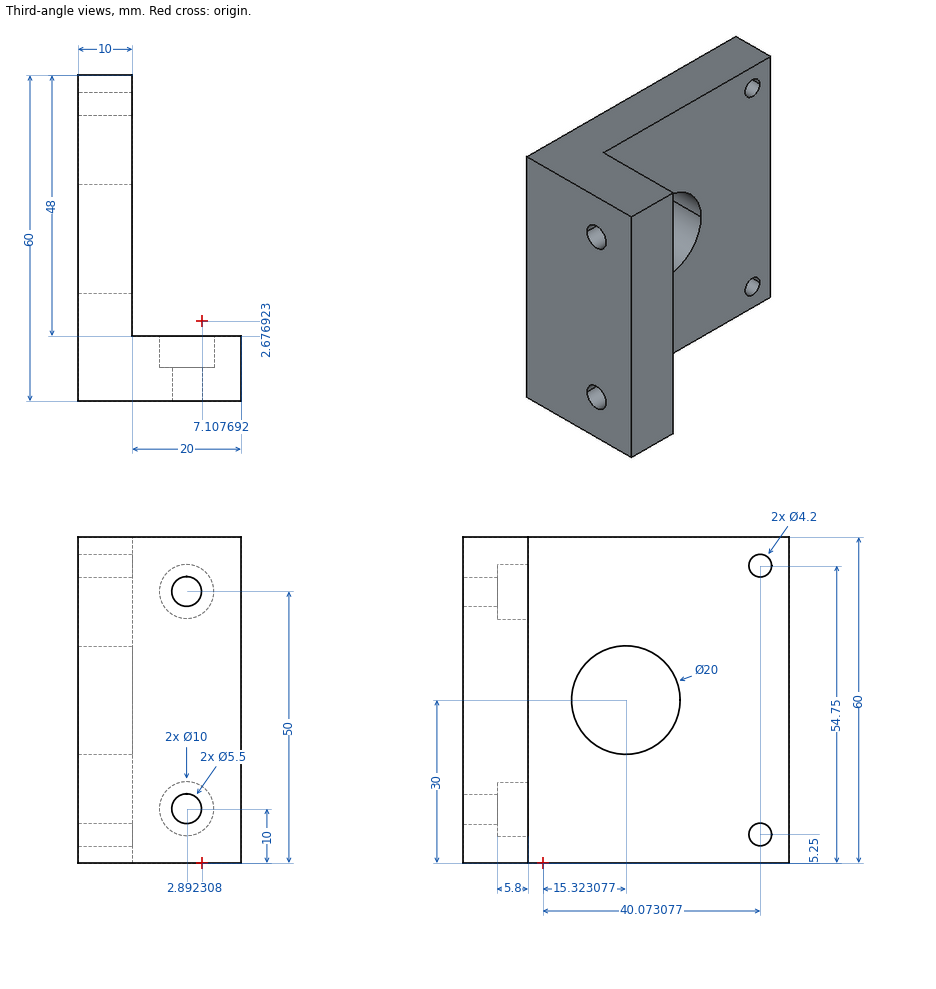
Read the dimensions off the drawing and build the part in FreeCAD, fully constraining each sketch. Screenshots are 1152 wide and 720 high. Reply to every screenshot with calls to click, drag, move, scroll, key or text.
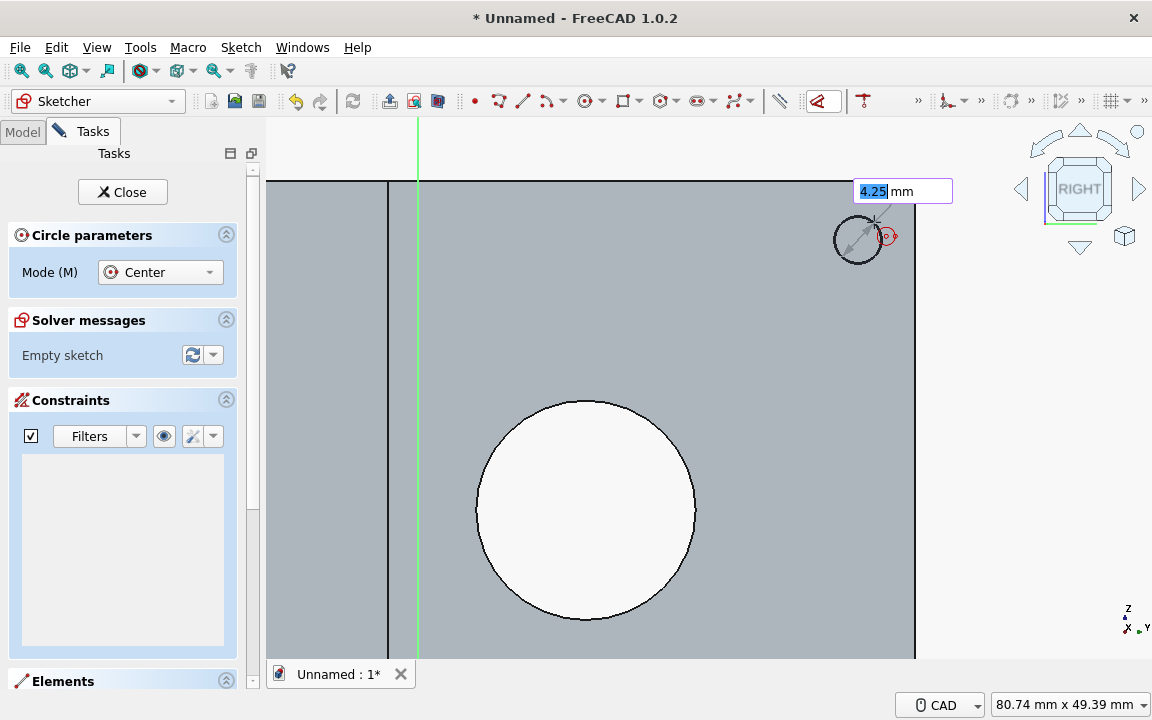
text(4.2)
key(Return)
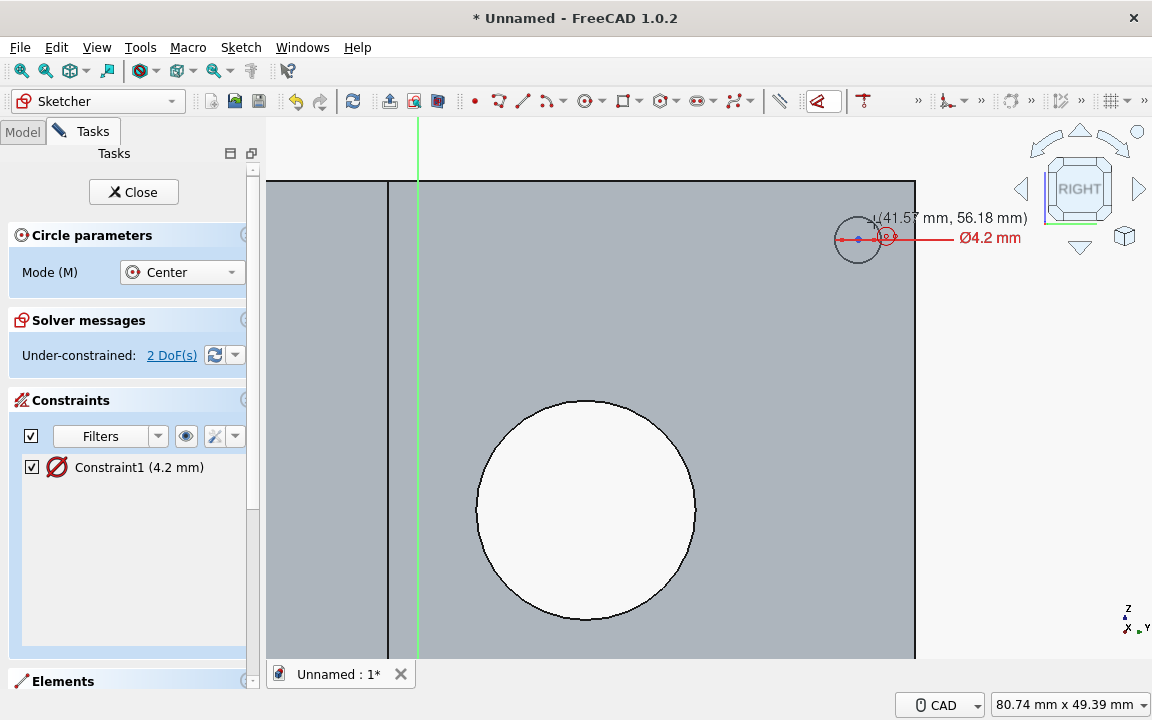
scroll(630, 218, down, 3)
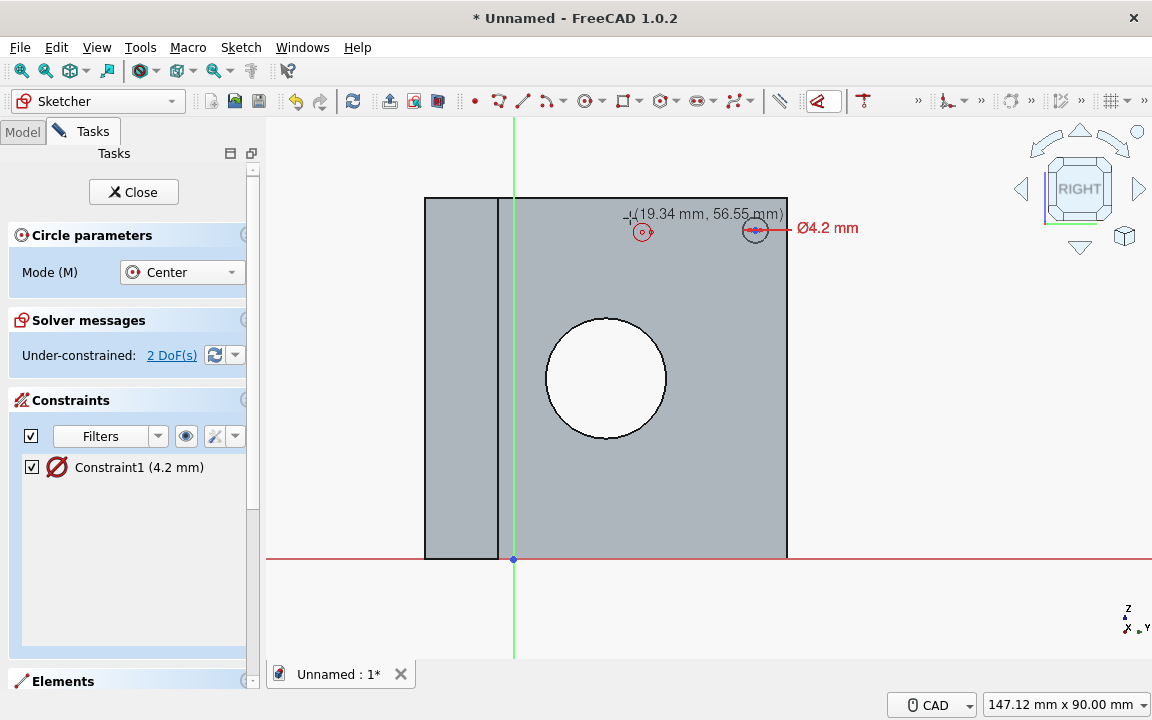
scroll(755, 528, up, 3)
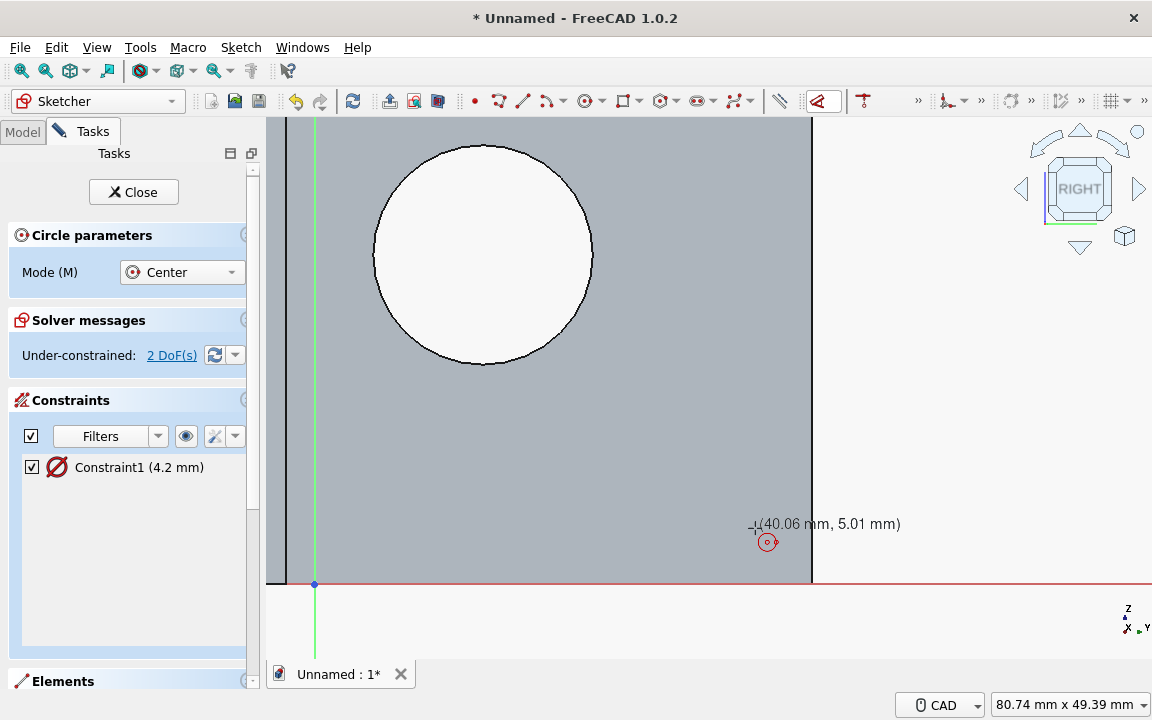
click(755, 527)
move(771, 510)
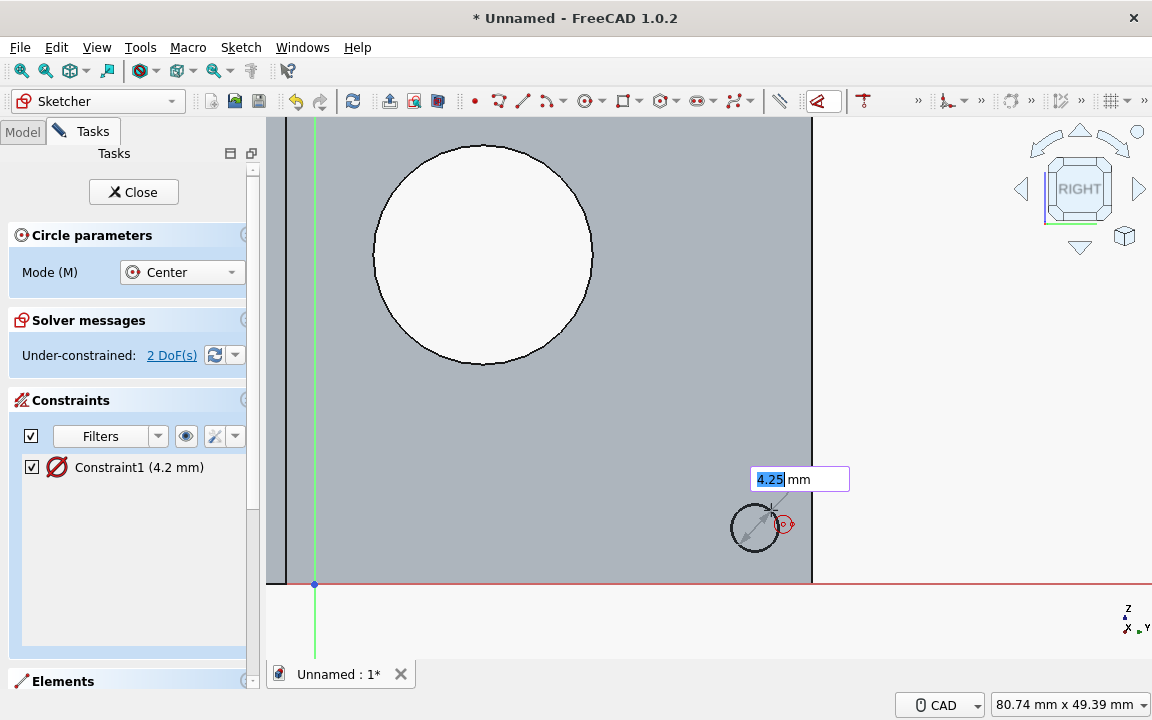
text(4.2)
key(Return)
key(Escape)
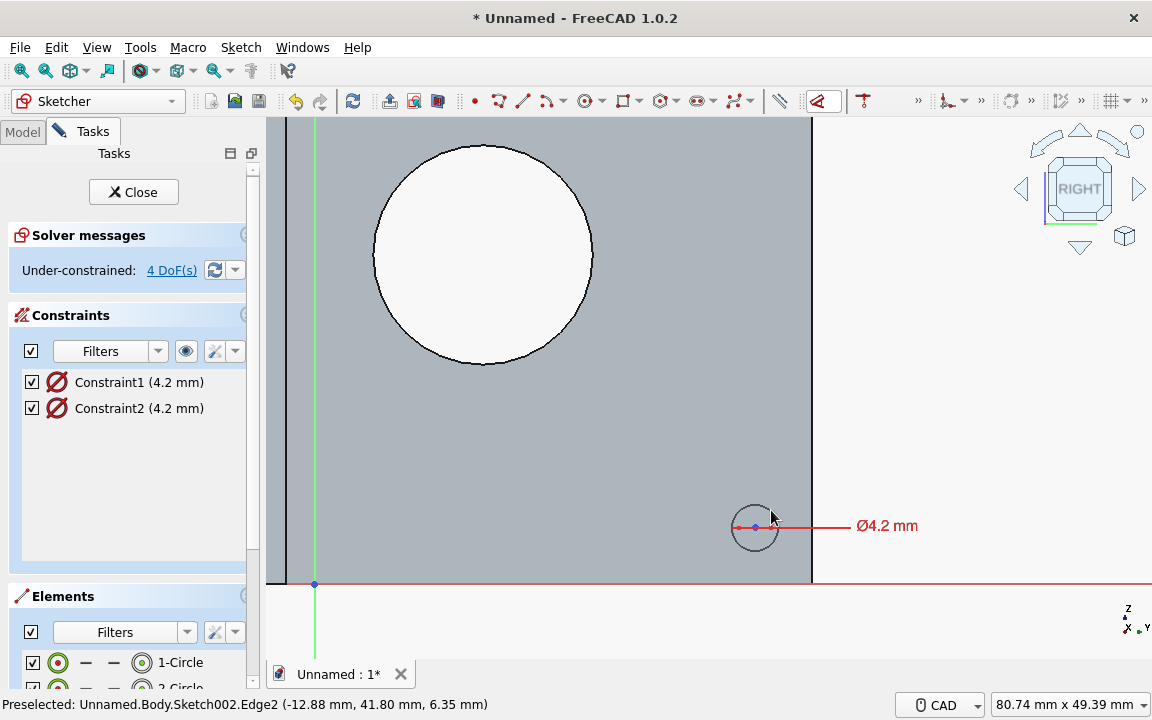
scroll(755, 529, down, 3)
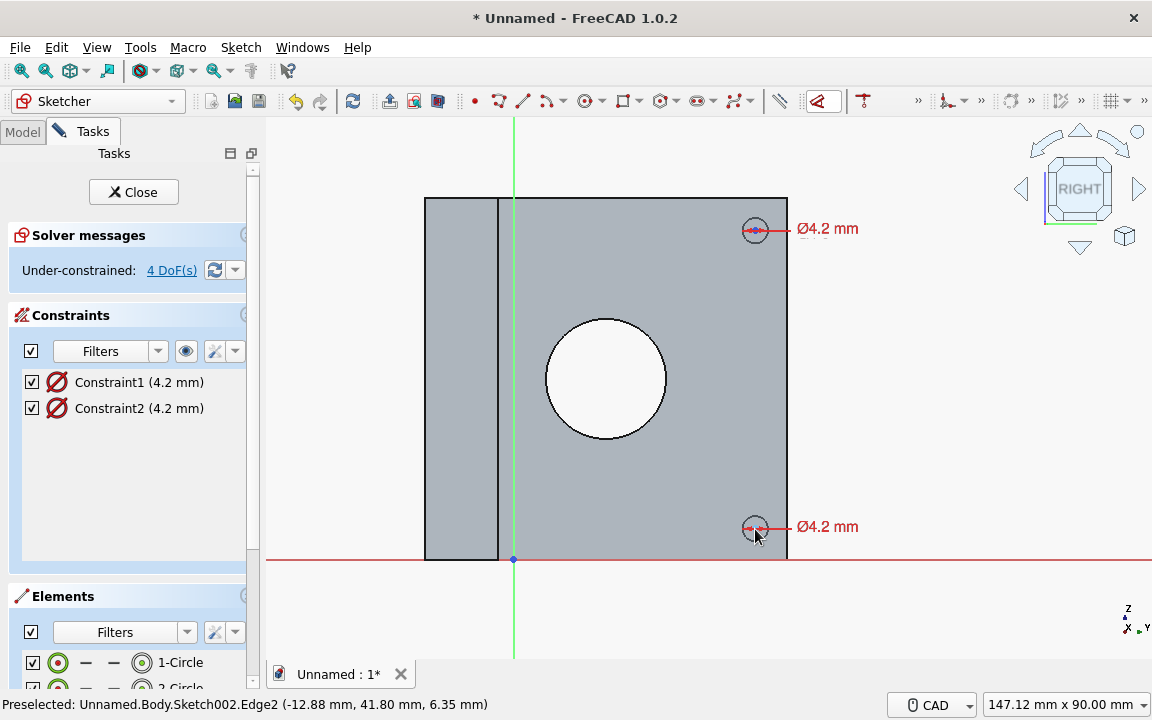
click(755, 231)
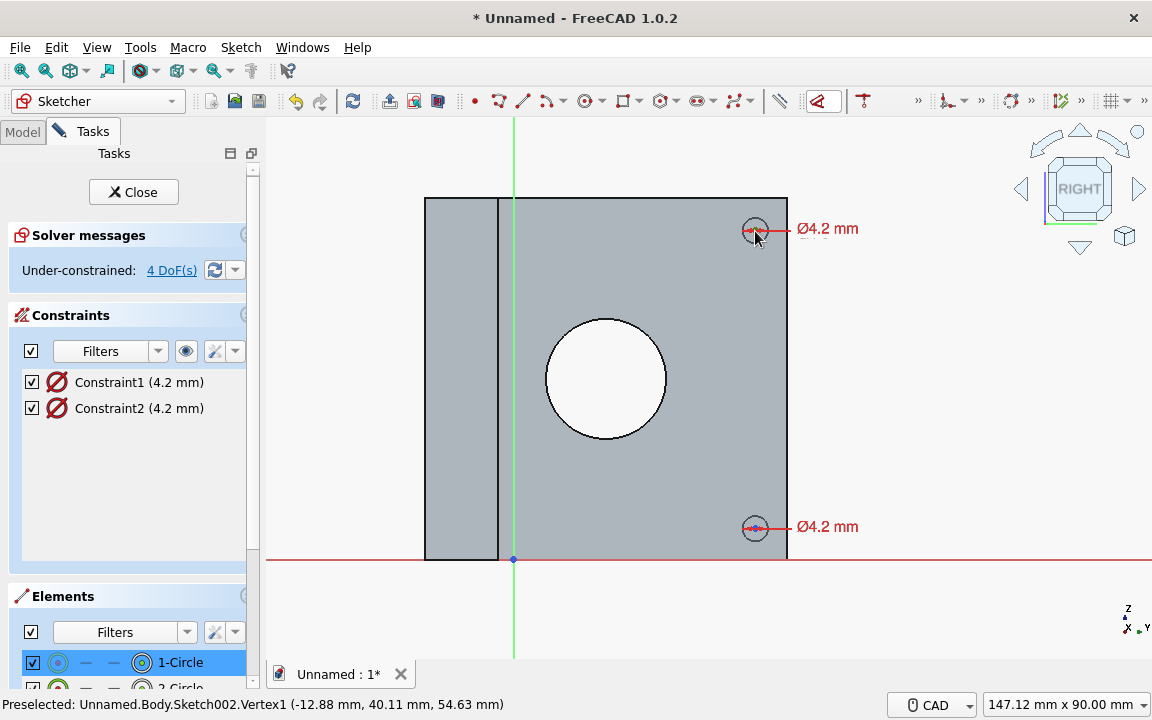
click(755, 529)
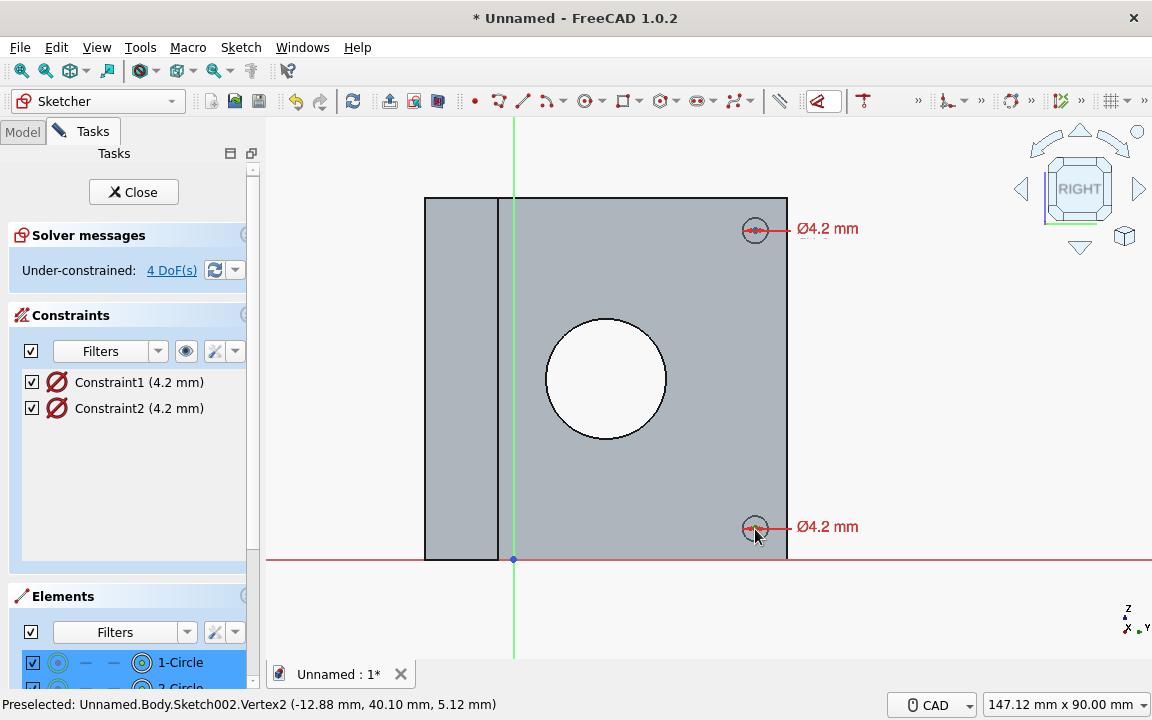
key(v)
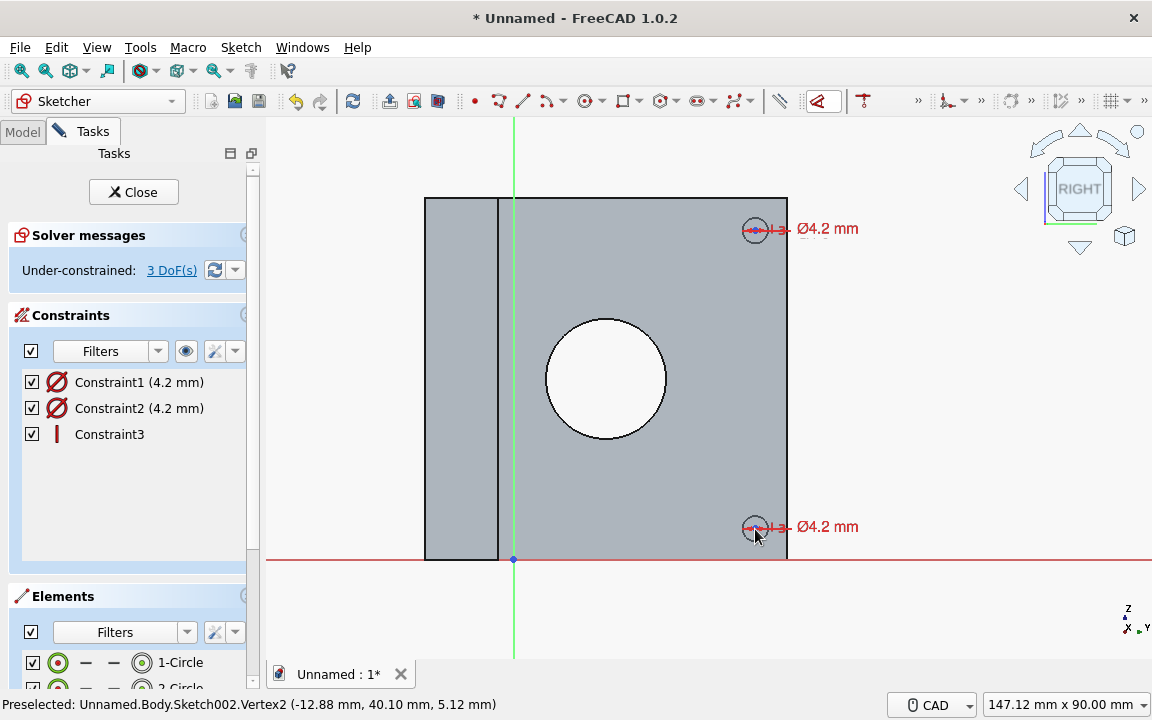
scroll(755, 529, up, 2)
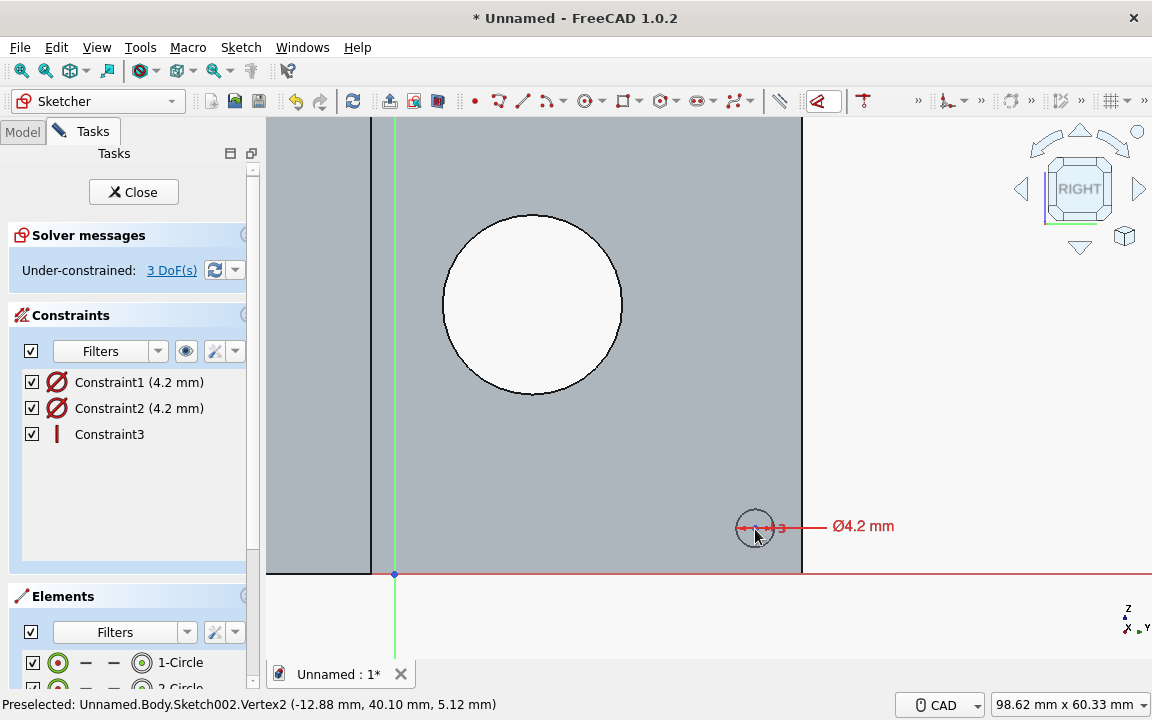
click(755, 528)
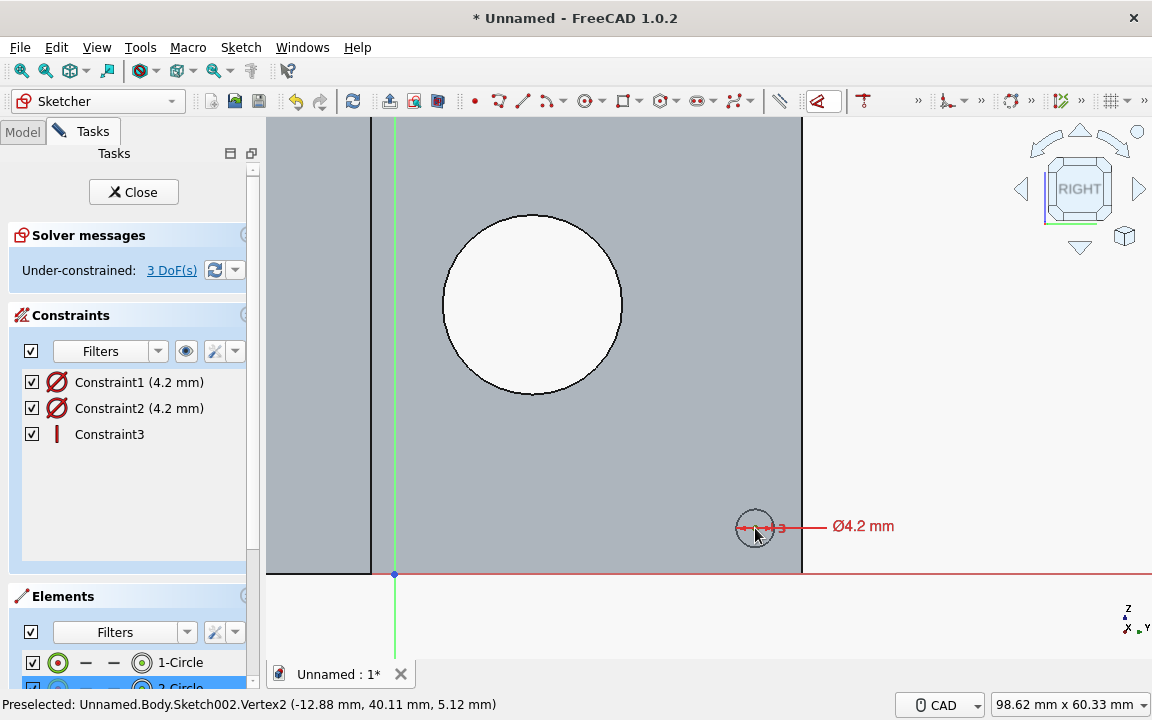
click(836, 102)